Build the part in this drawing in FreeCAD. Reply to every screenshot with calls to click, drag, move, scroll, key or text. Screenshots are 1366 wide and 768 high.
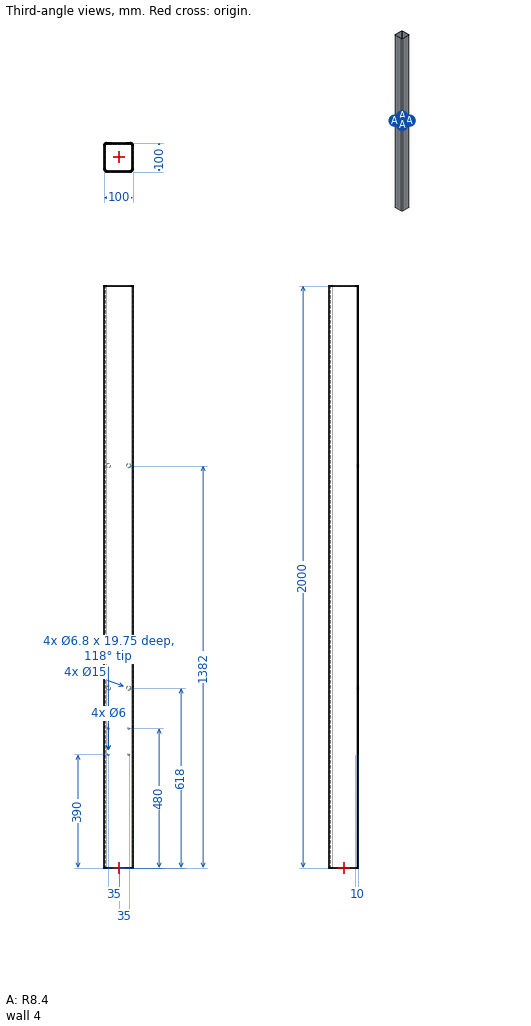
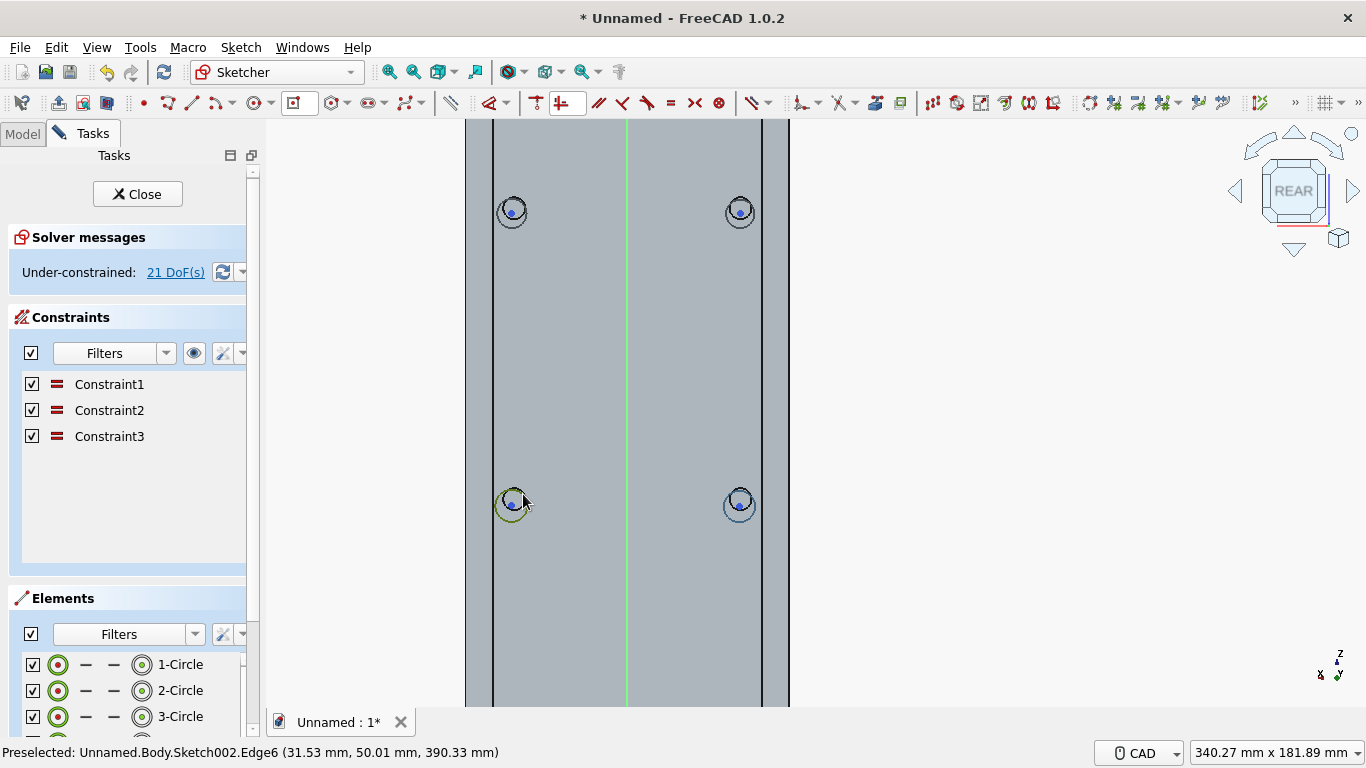
click(522, 203)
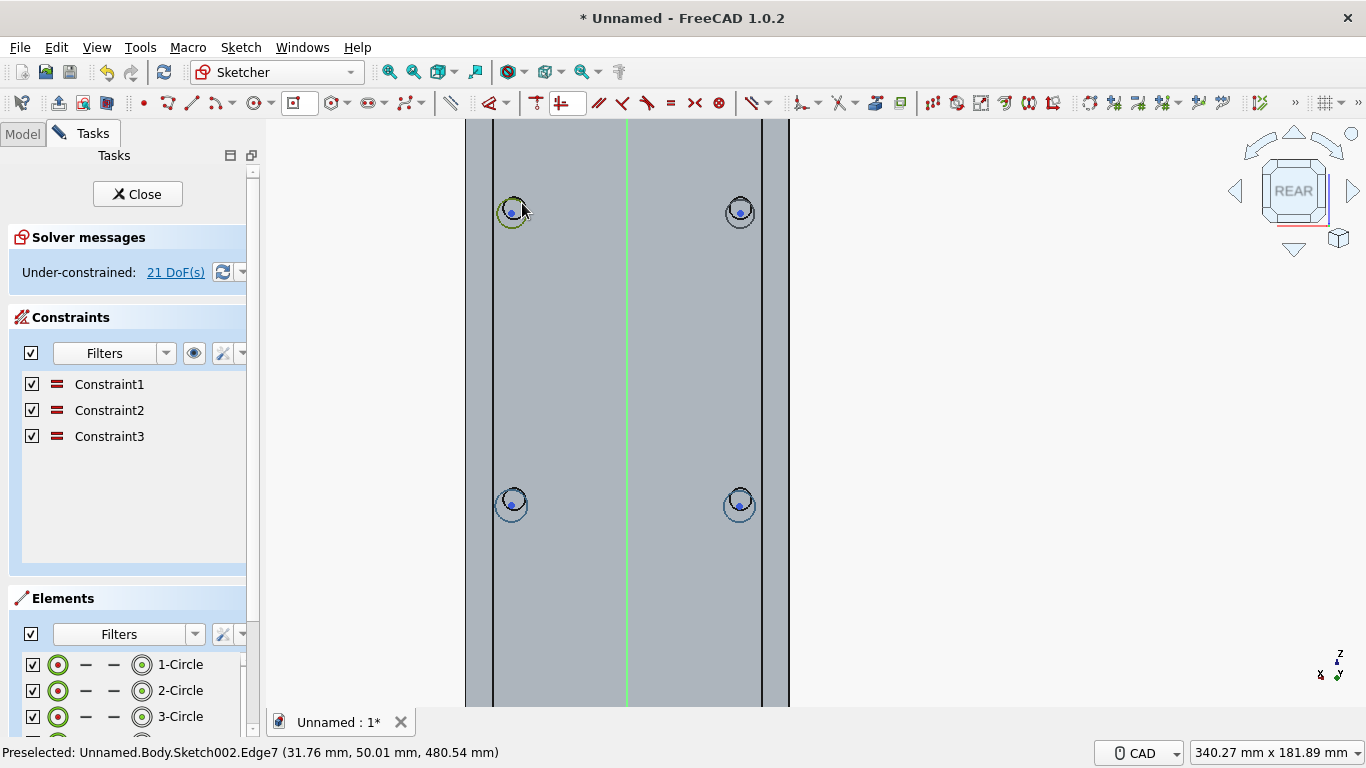
click(750, 204)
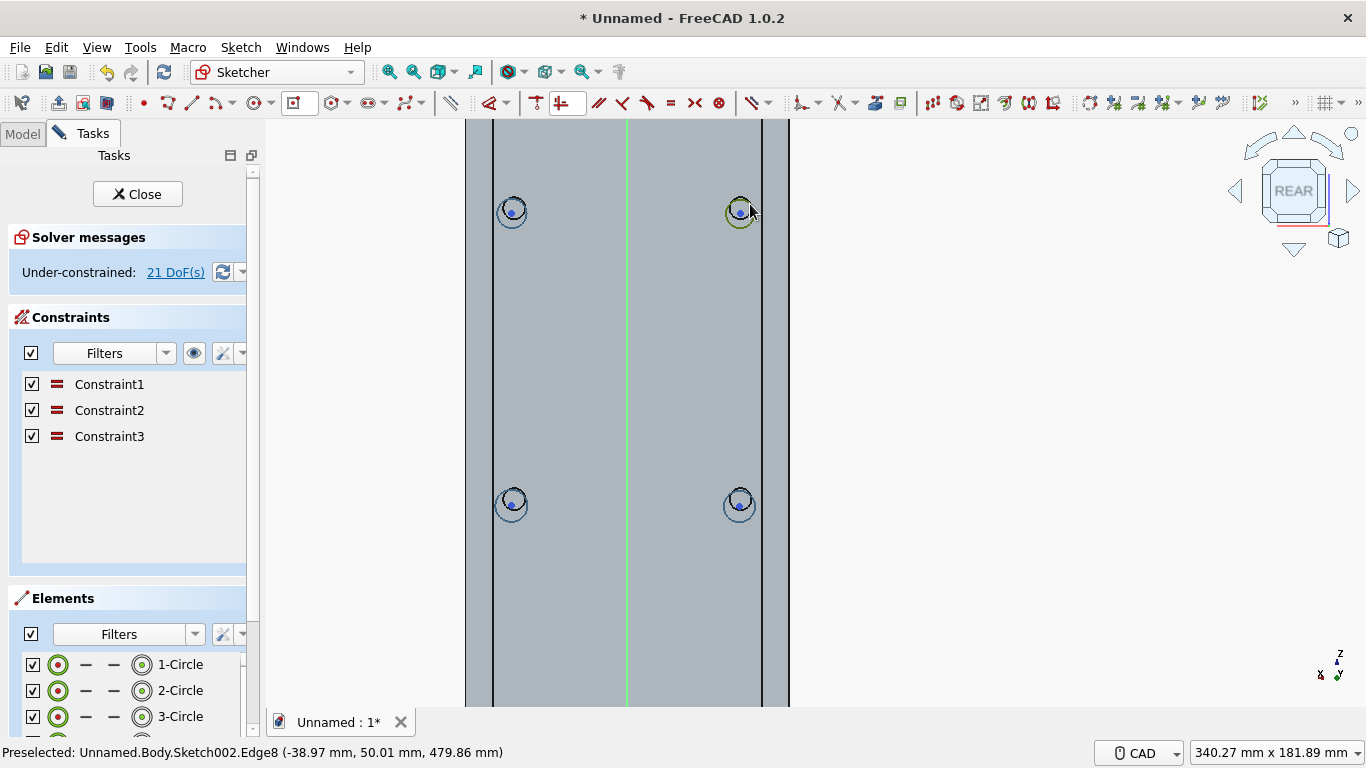
click(672, 104)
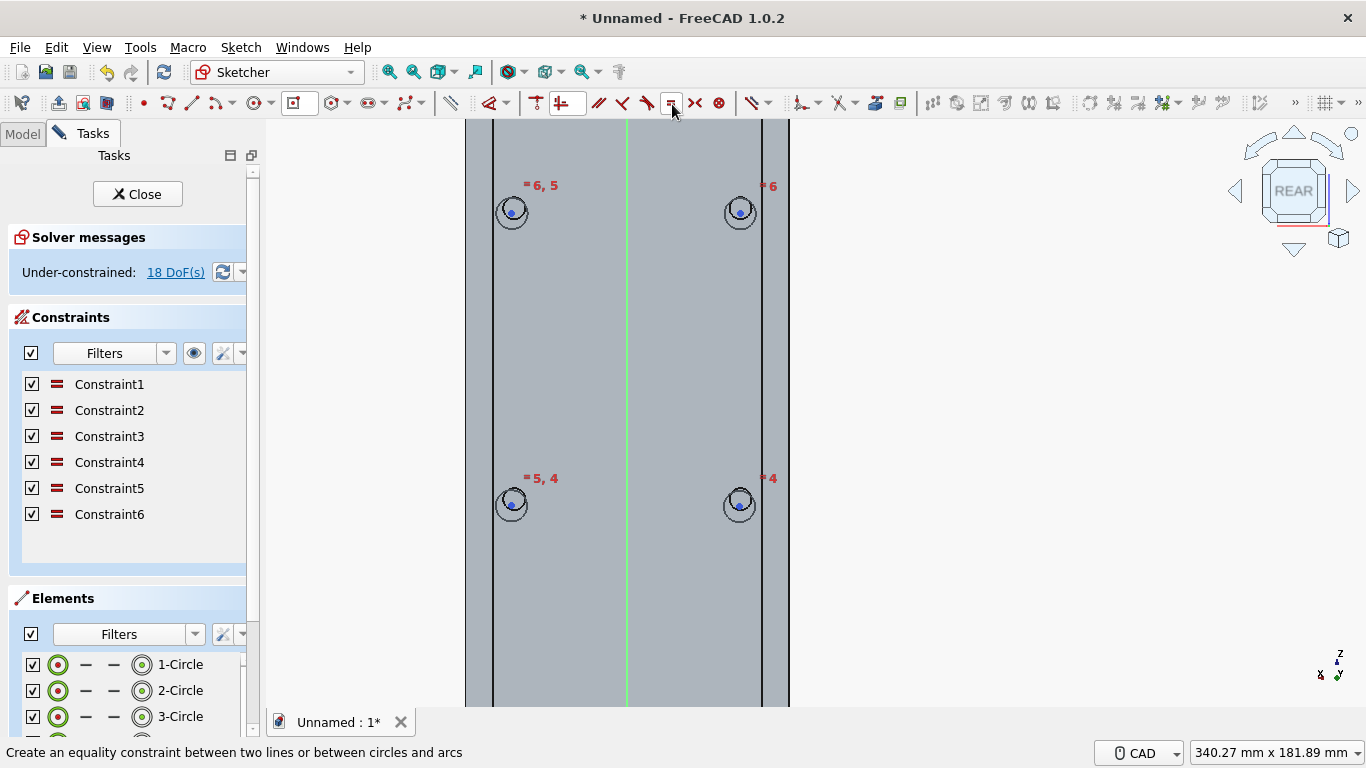
scroll(759, 503, down, 12)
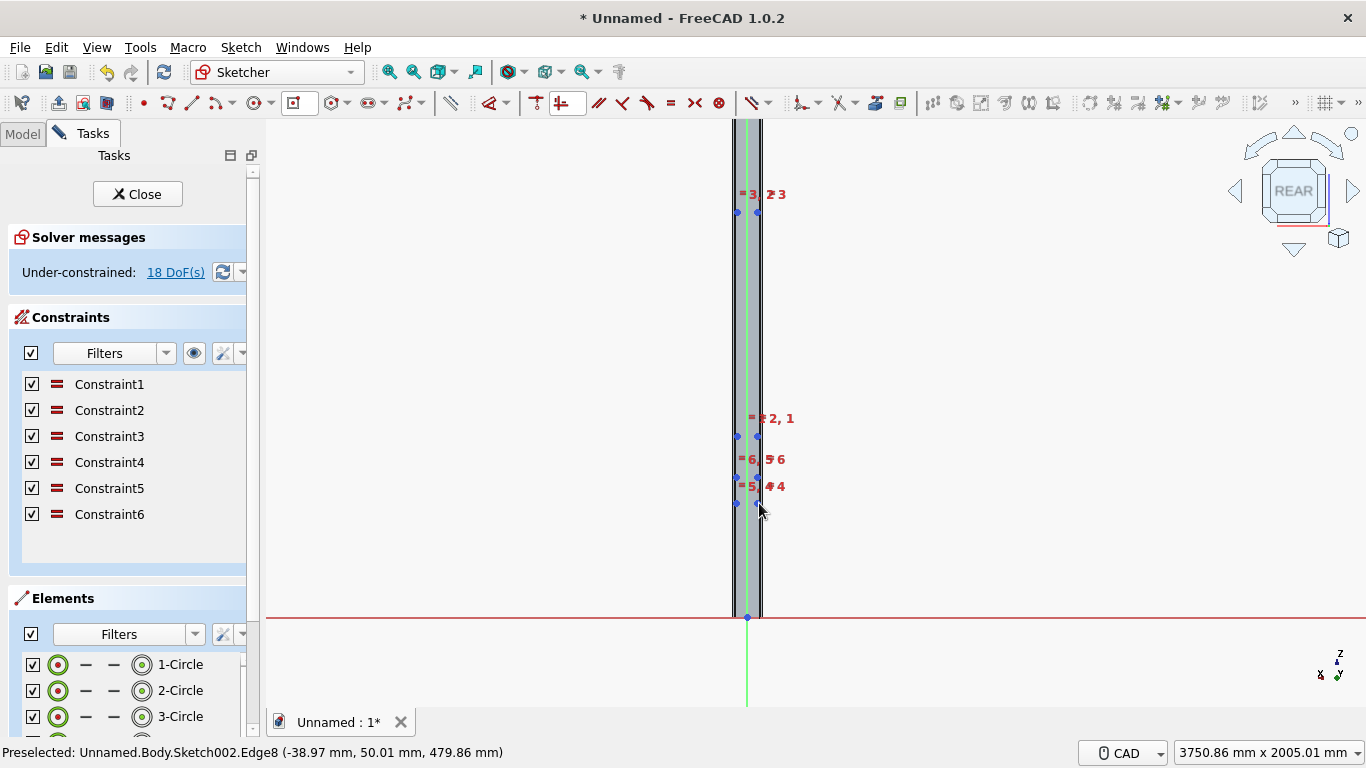
click(737, 437)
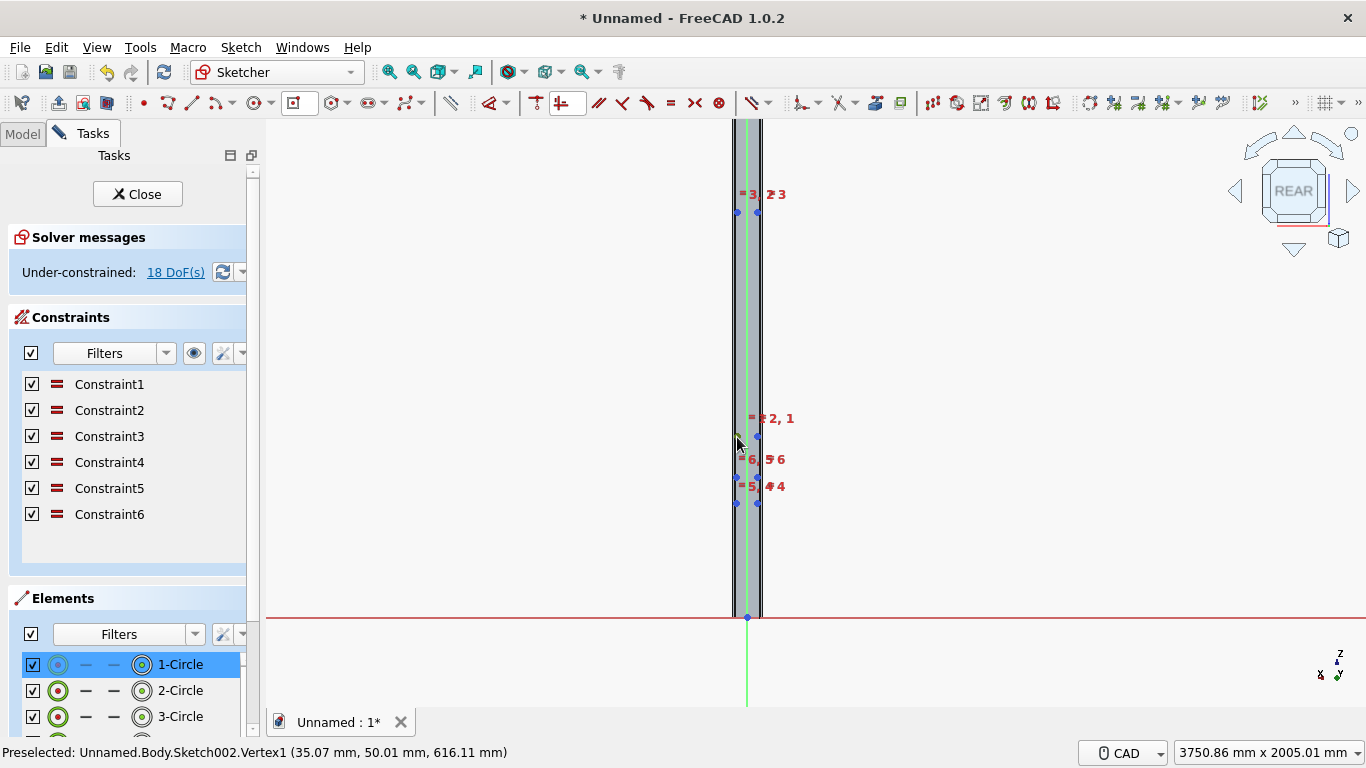
click(758, 437)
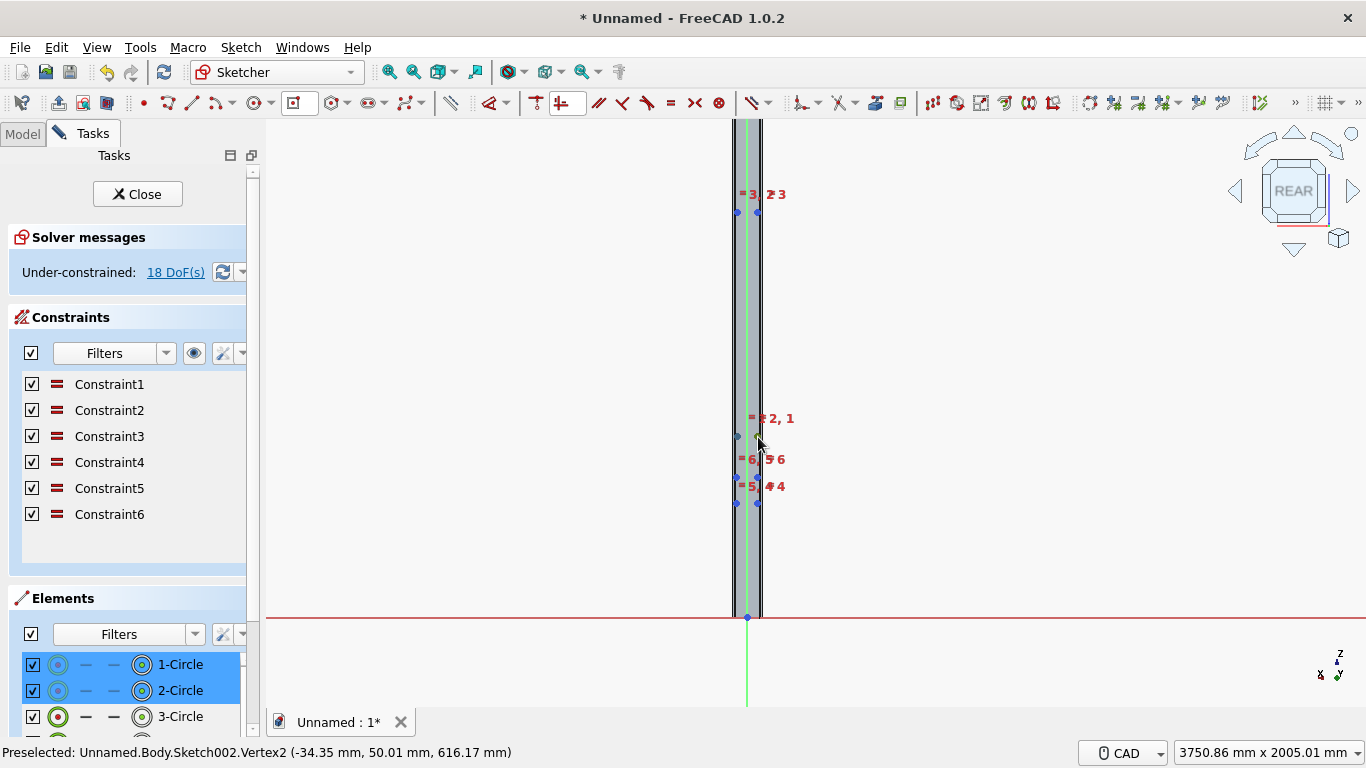
click(580, 104)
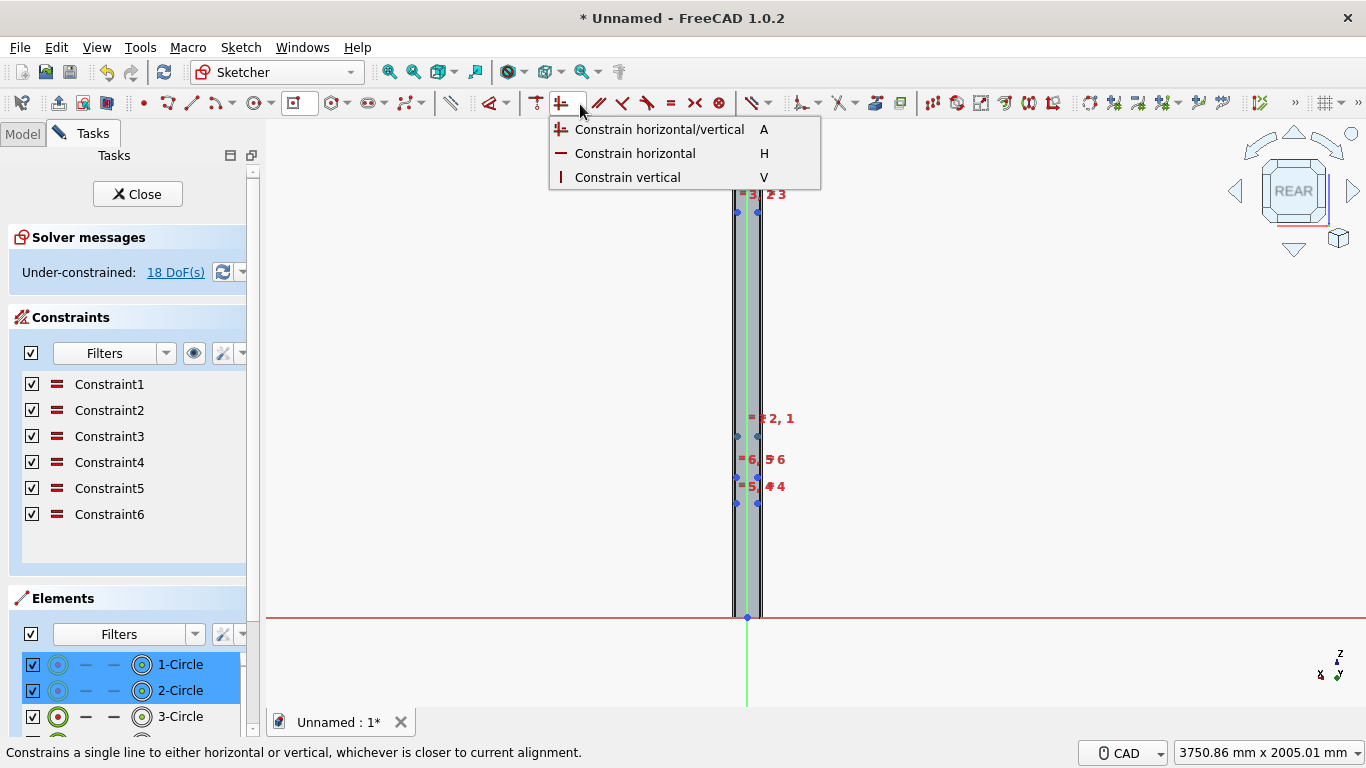
click(685, 153)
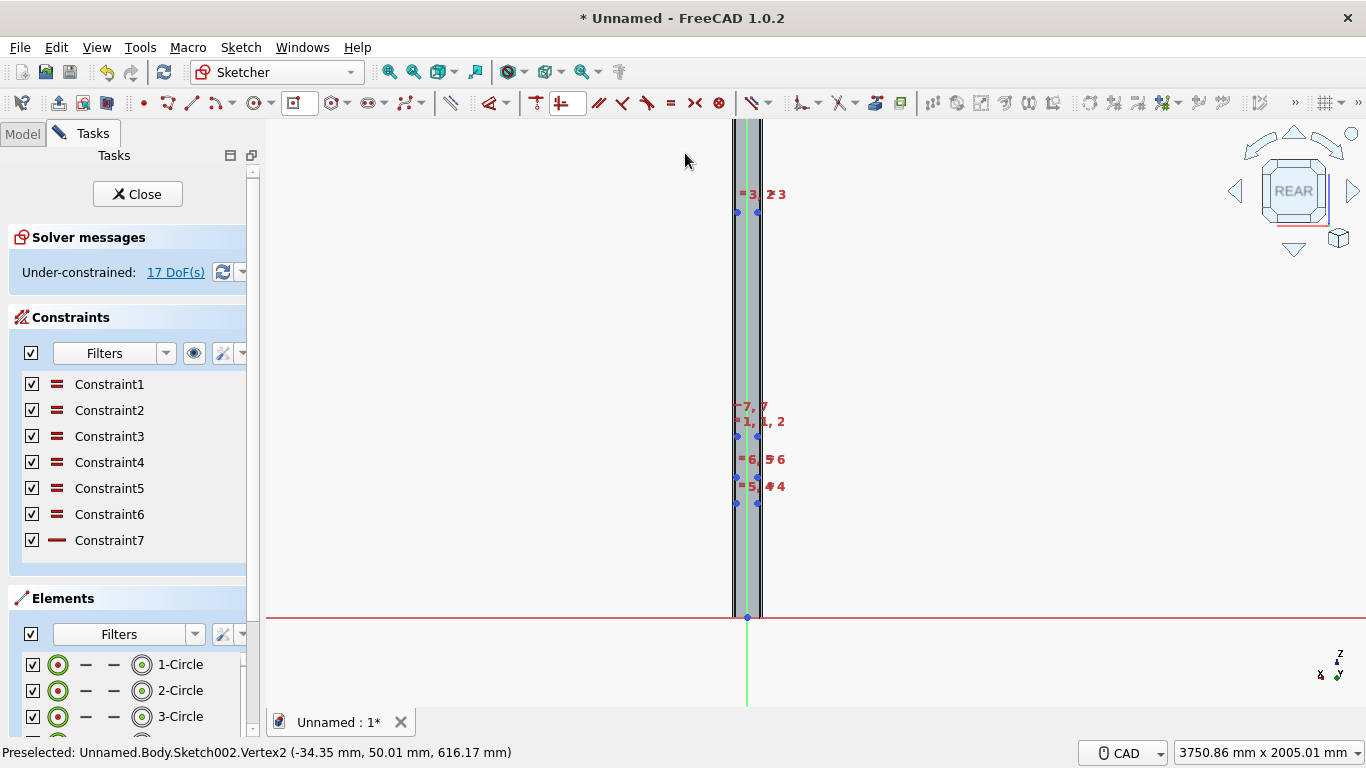
click(737, 437)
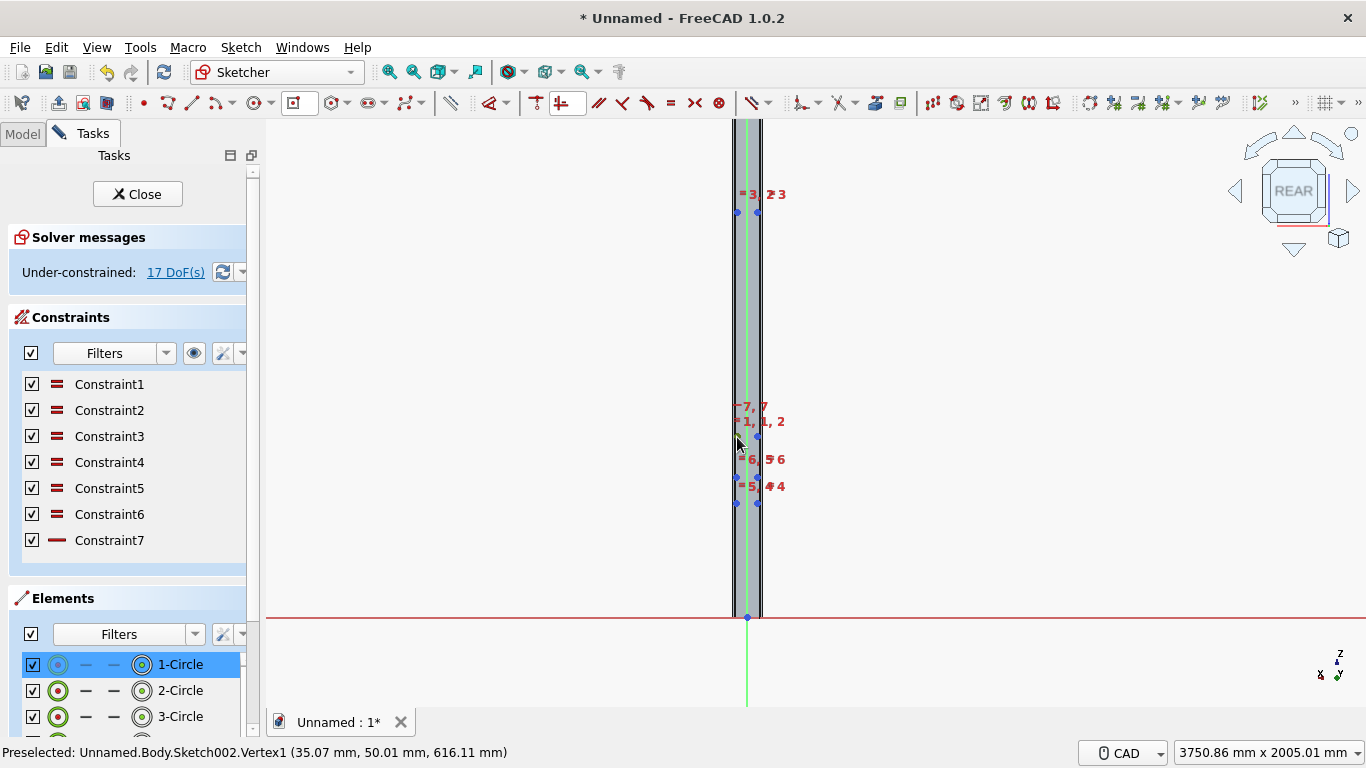
click(737, 213)